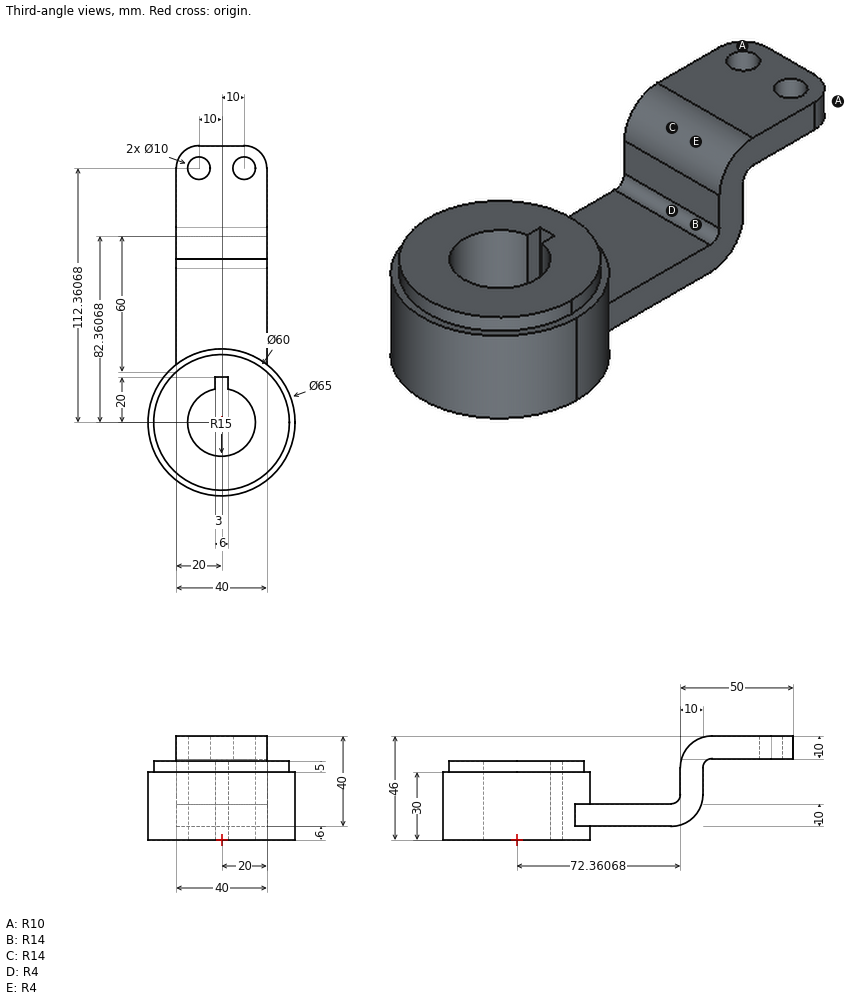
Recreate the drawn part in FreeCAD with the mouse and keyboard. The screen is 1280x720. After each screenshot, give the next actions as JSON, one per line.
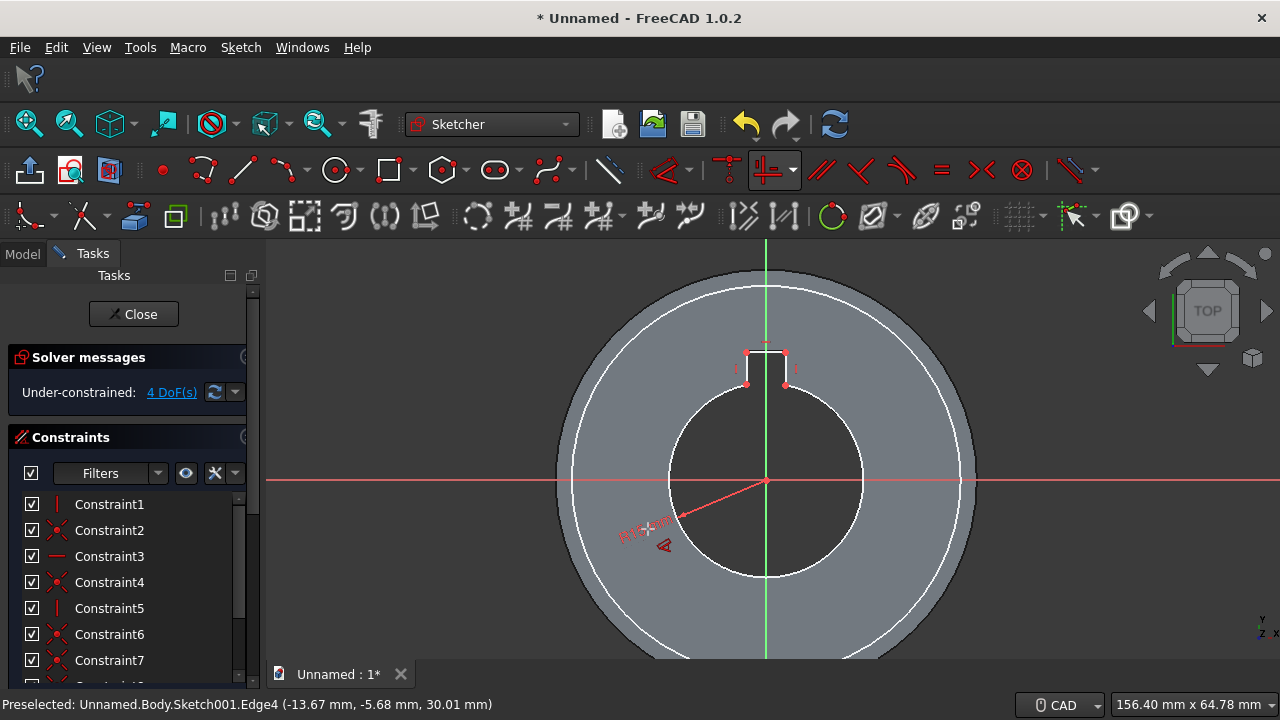
{"action": "left_click", "coordinate": [903, 342]}
{"action": "left_click", "coordinate": [926, 319]}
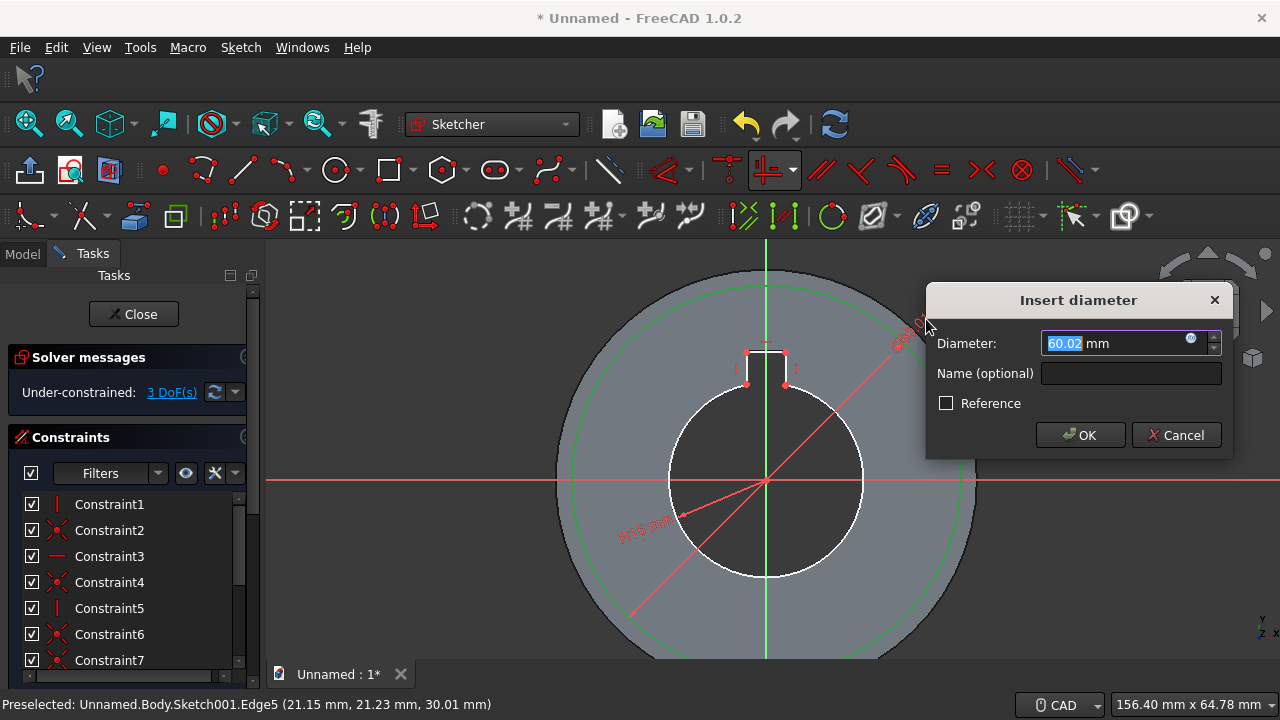
{"action": "type", "text": "60"}
{"action": "key", "text": "Return"}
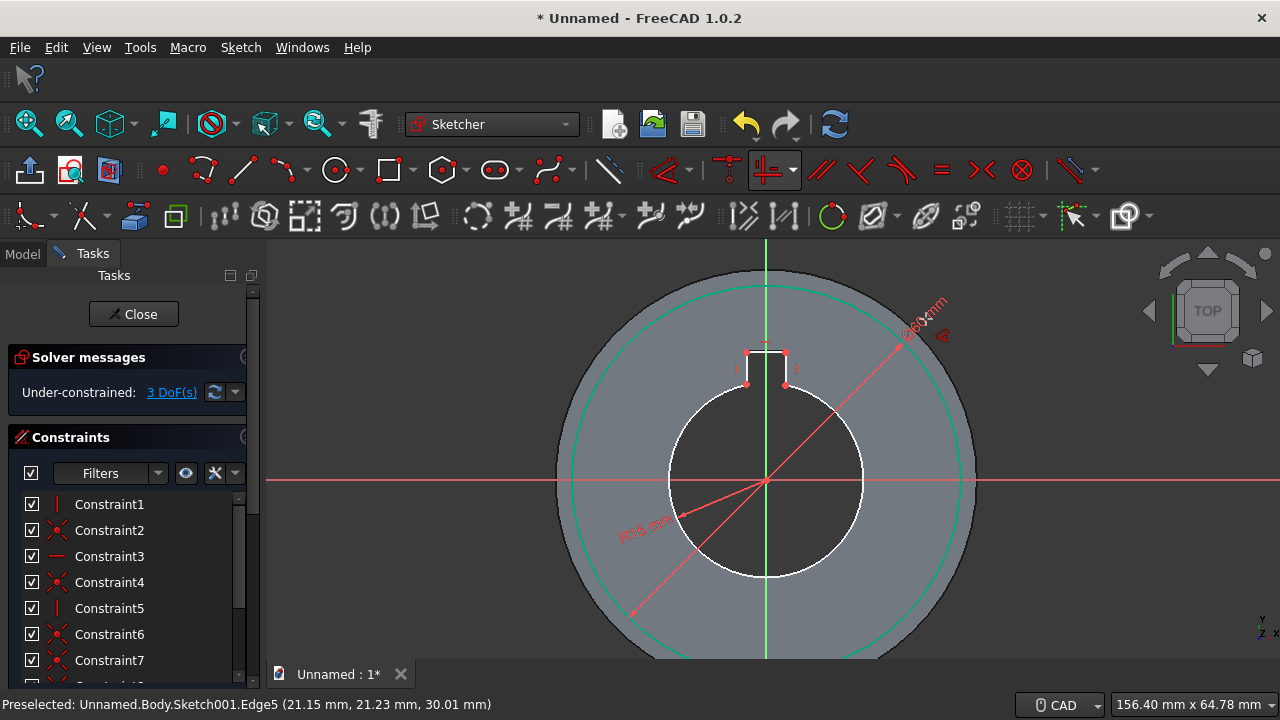
{"action": "left_click", "coordinate": [762, 352]}
{"action": "left_click", "coordinate": [753, 318]}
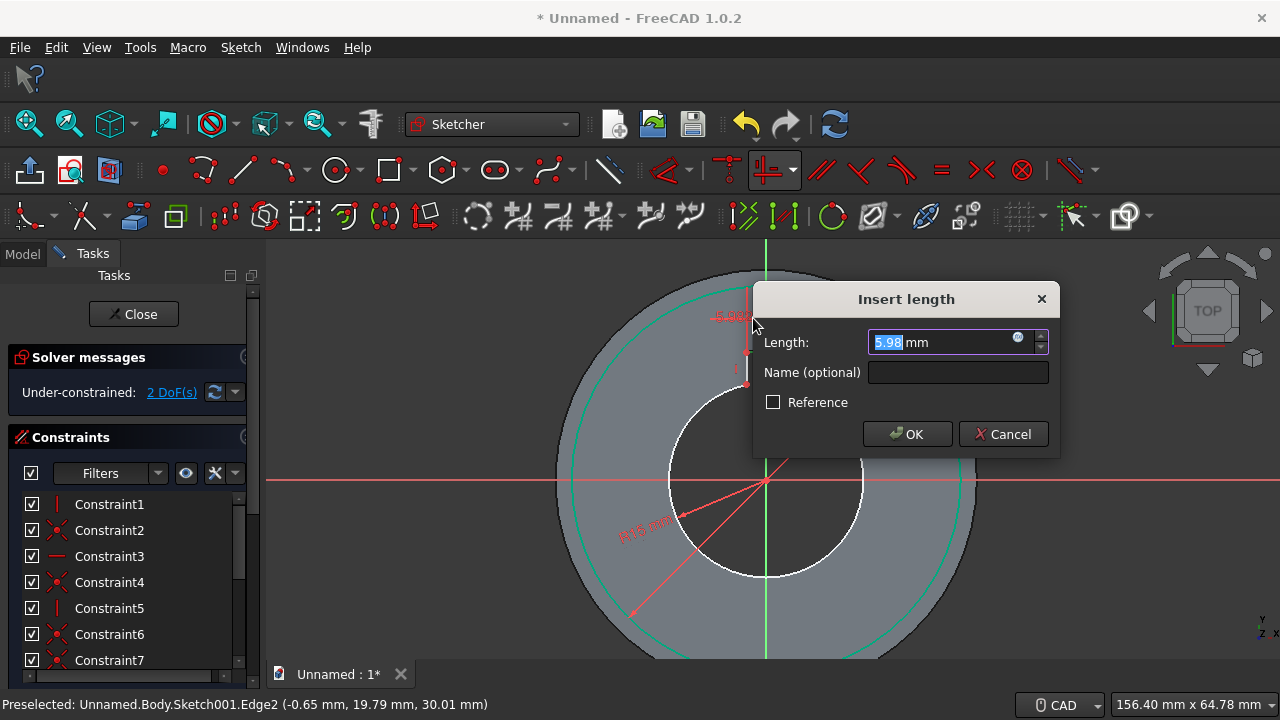
{"action": "type", "text": "6"}
{"action": "key", "text": "Return"}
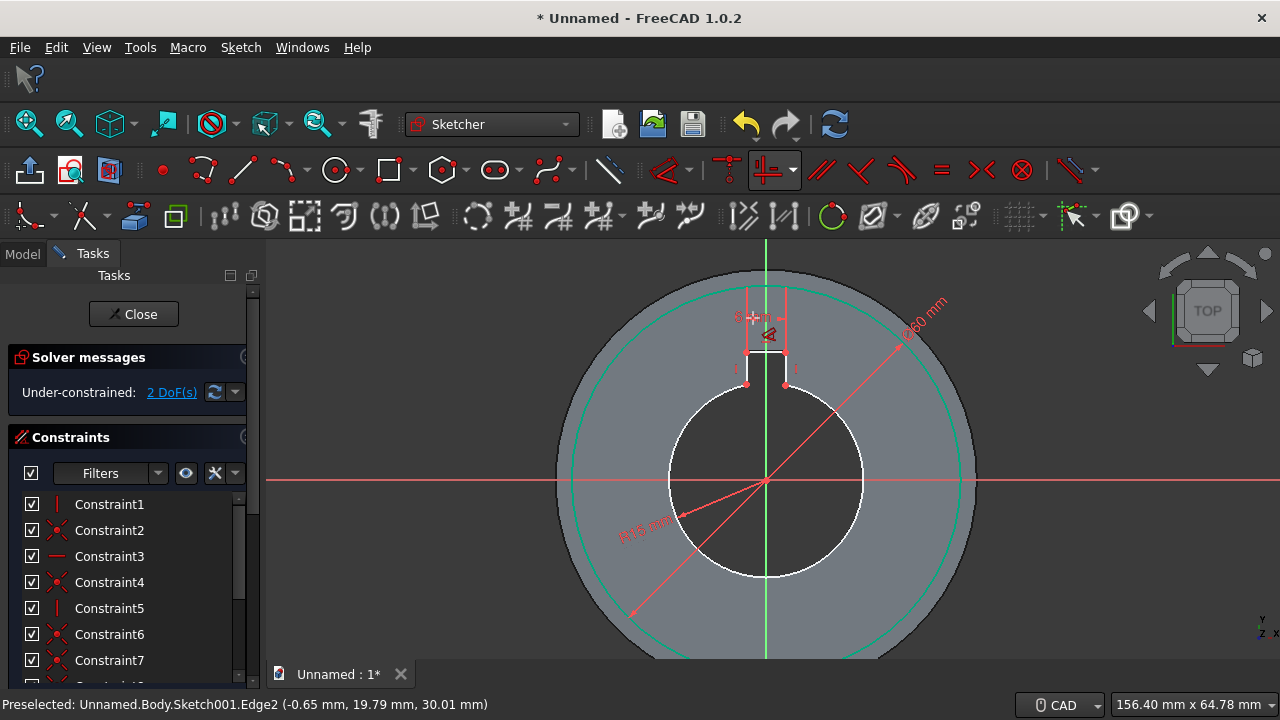
{"action": "scroll", "coordinate": [747, 385], "scroll_direction": "up", "scroll_amount": 4}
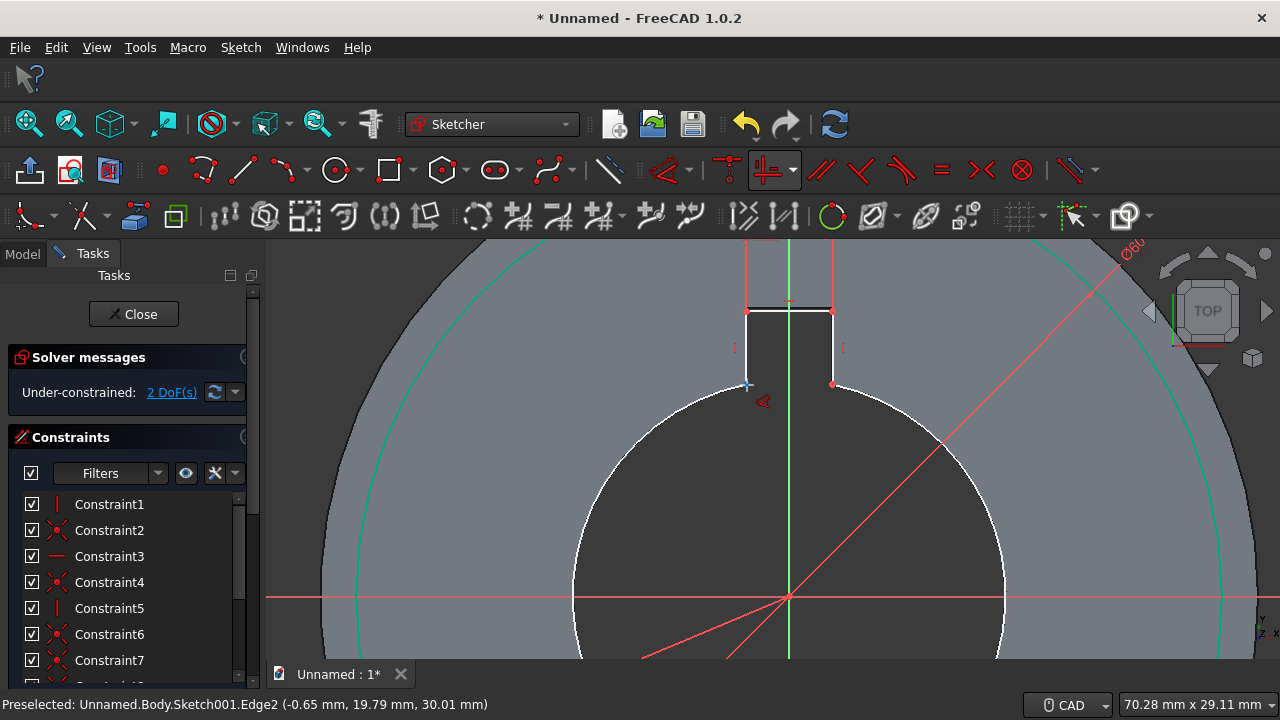
{"action": "left_click", "coordinate": [746, 385]}
{"action": "left_click", "coordinate": [768, 351]}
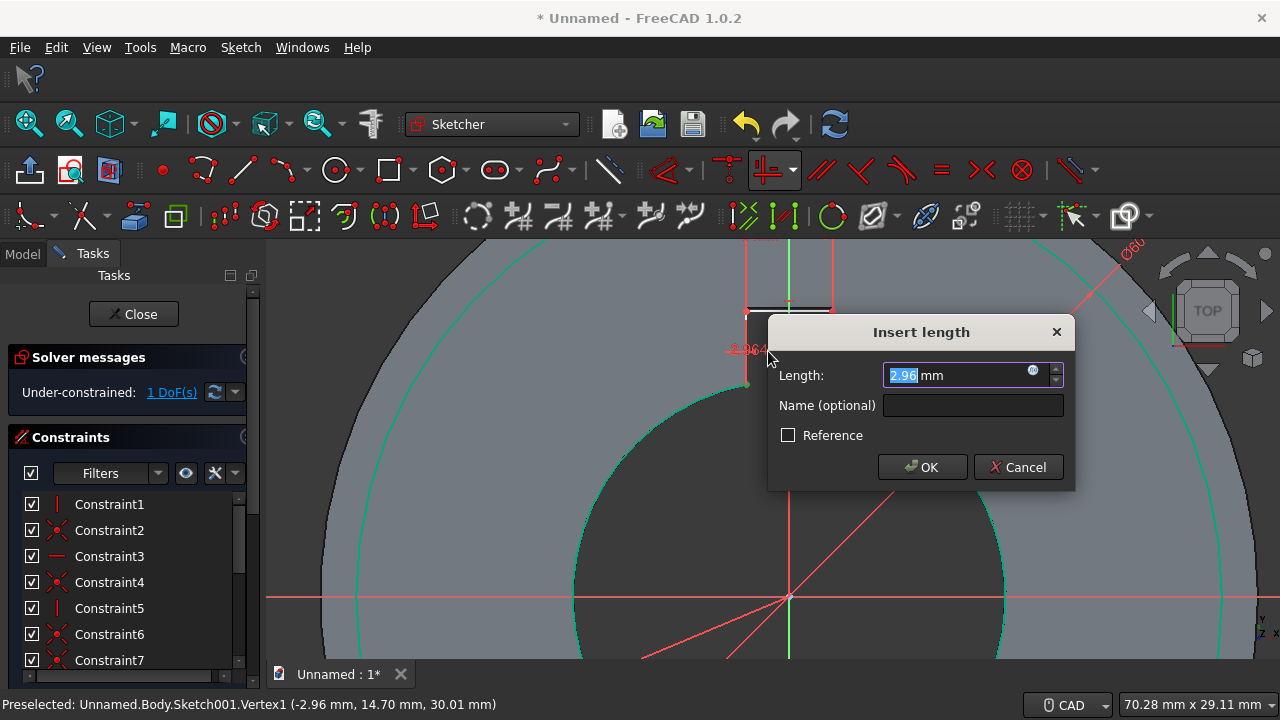
{"action": "type", "text": "3"}
{"action": "key", "text": "Return"}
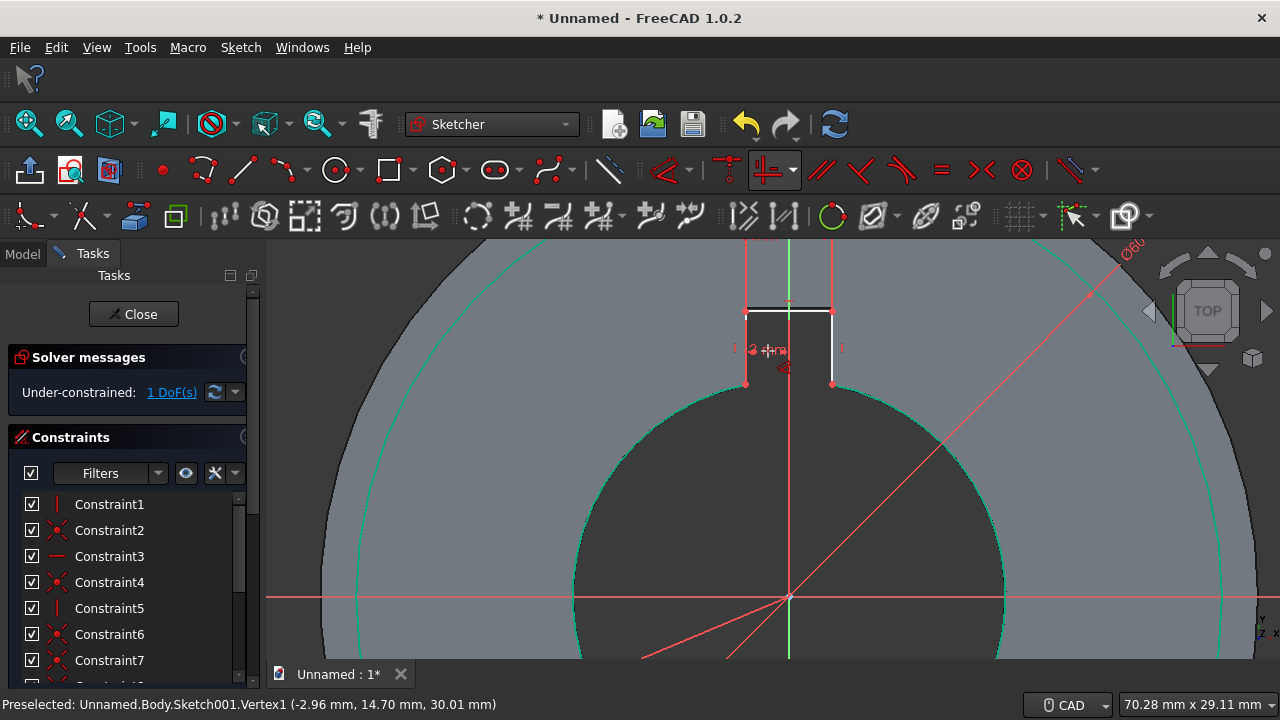
{"action": "left_click", "coordinate": [746, 311]}
{"action": "left_click", "coordinate": [712, 454]}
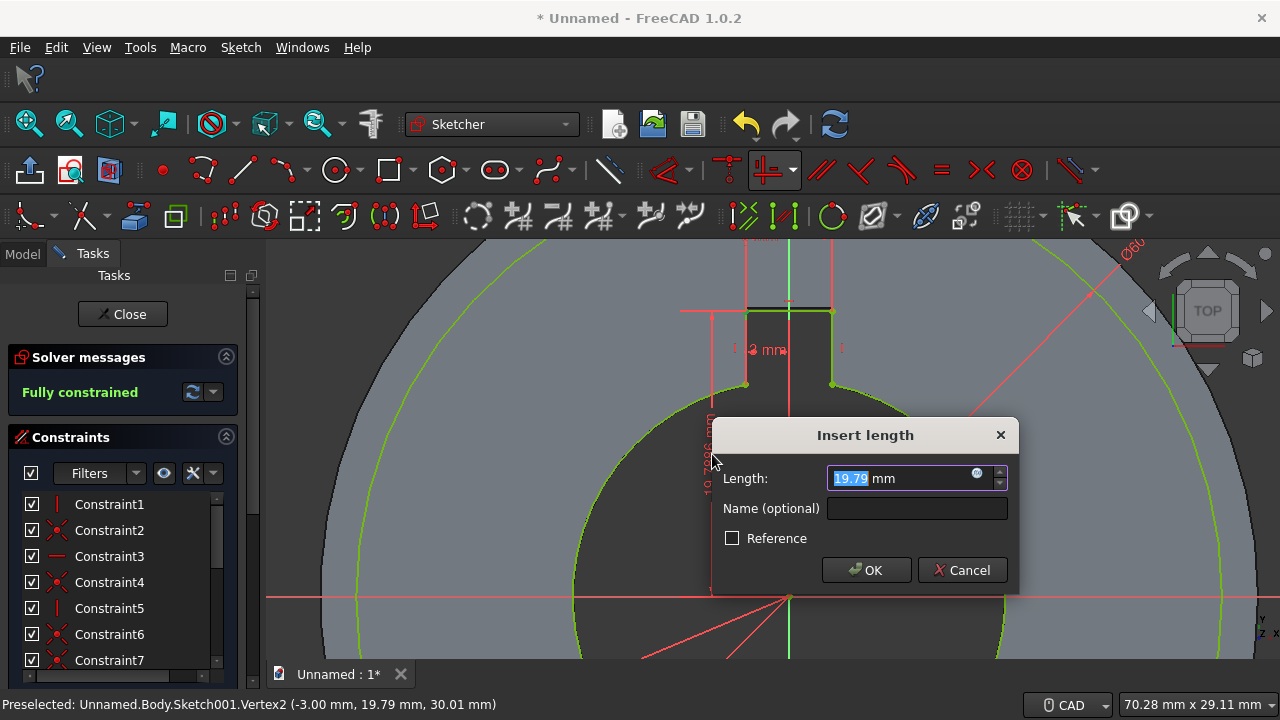
{"action": "type", "text": "20"}
{"action": "key", "text": "Return"}
{"action": "key", "text": "Escape"}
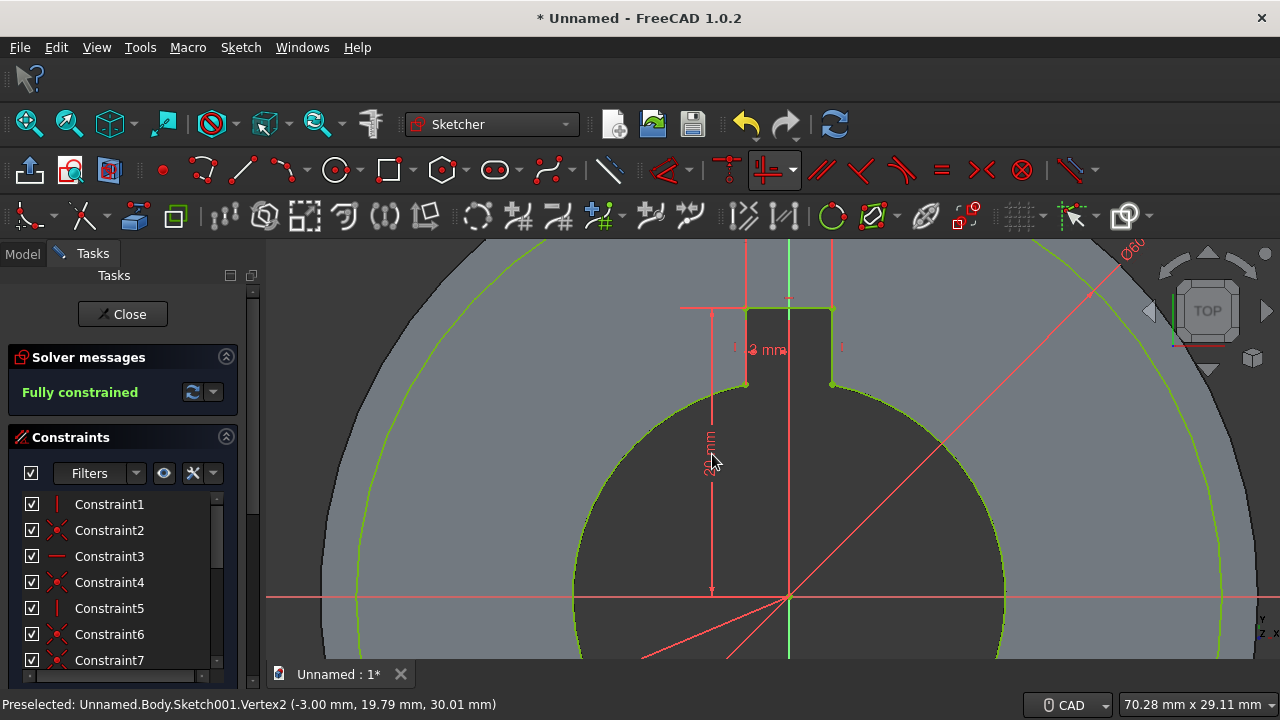
{"action": "left_click", "coordinate": [123, 314]}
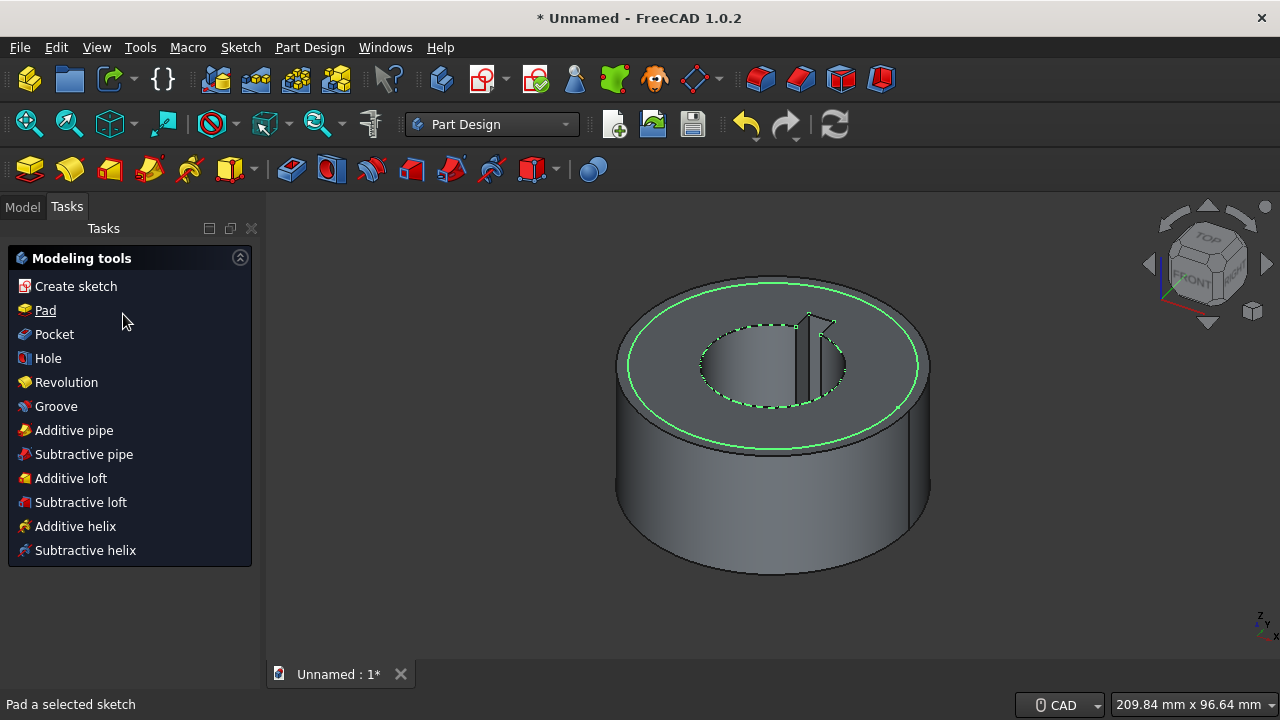
{"action": "left_click", "coordinate": [30, 170]}